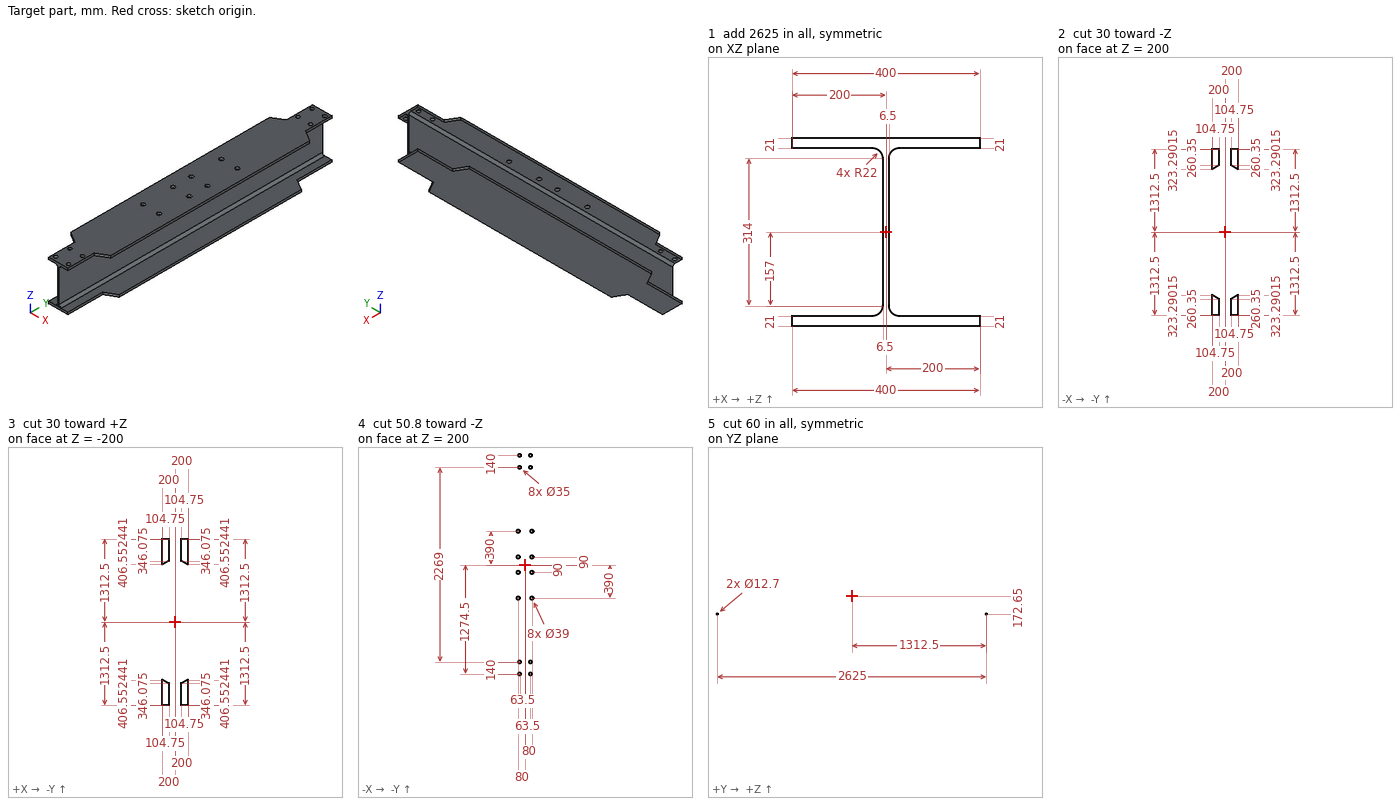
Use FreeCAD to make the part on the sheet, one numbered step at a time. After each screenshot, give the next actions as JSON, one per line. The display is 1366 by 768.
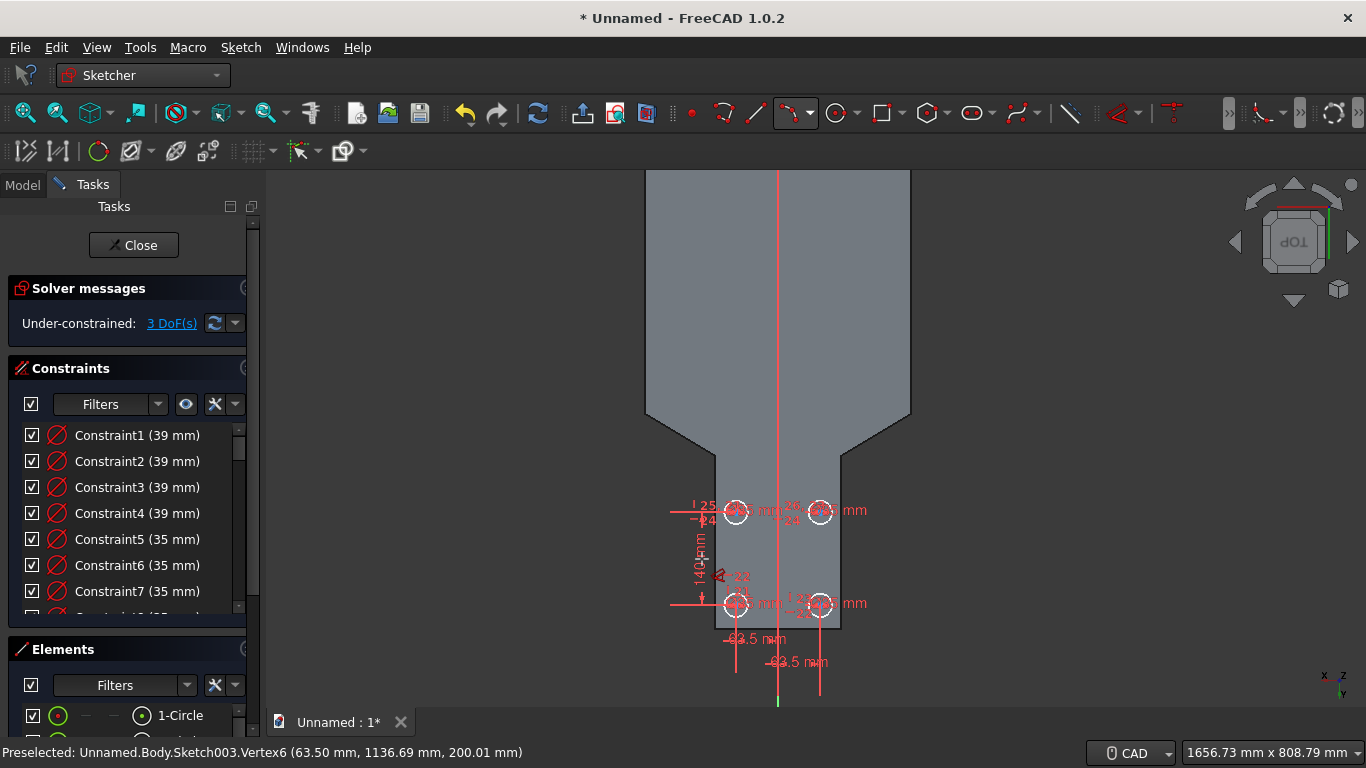
{"action": "scroll", "coordinate": [740, 611], "scroll_direction": "down", "scroll_amount": 8}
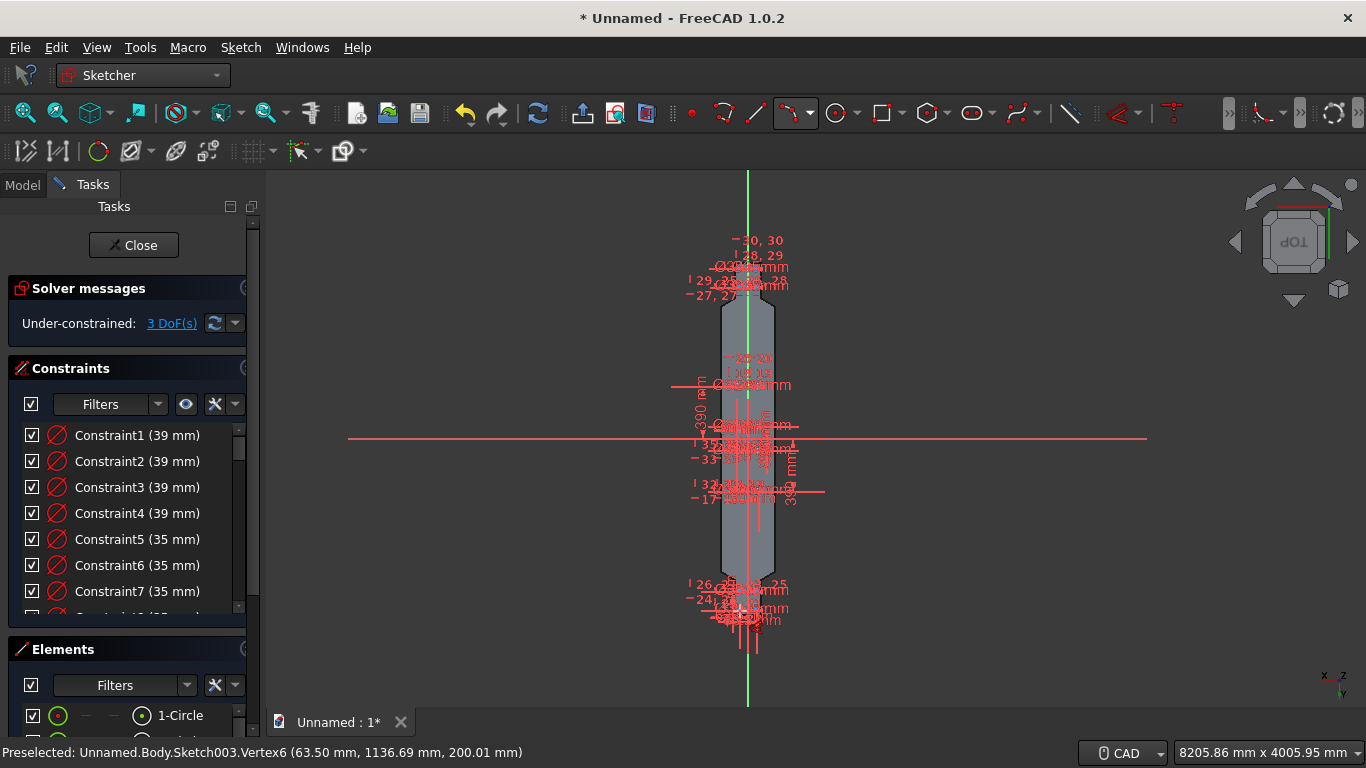
{"action": "scroll", "coordinate": [740, 288], "scroll_direction": "up", "scroll_amount": 4}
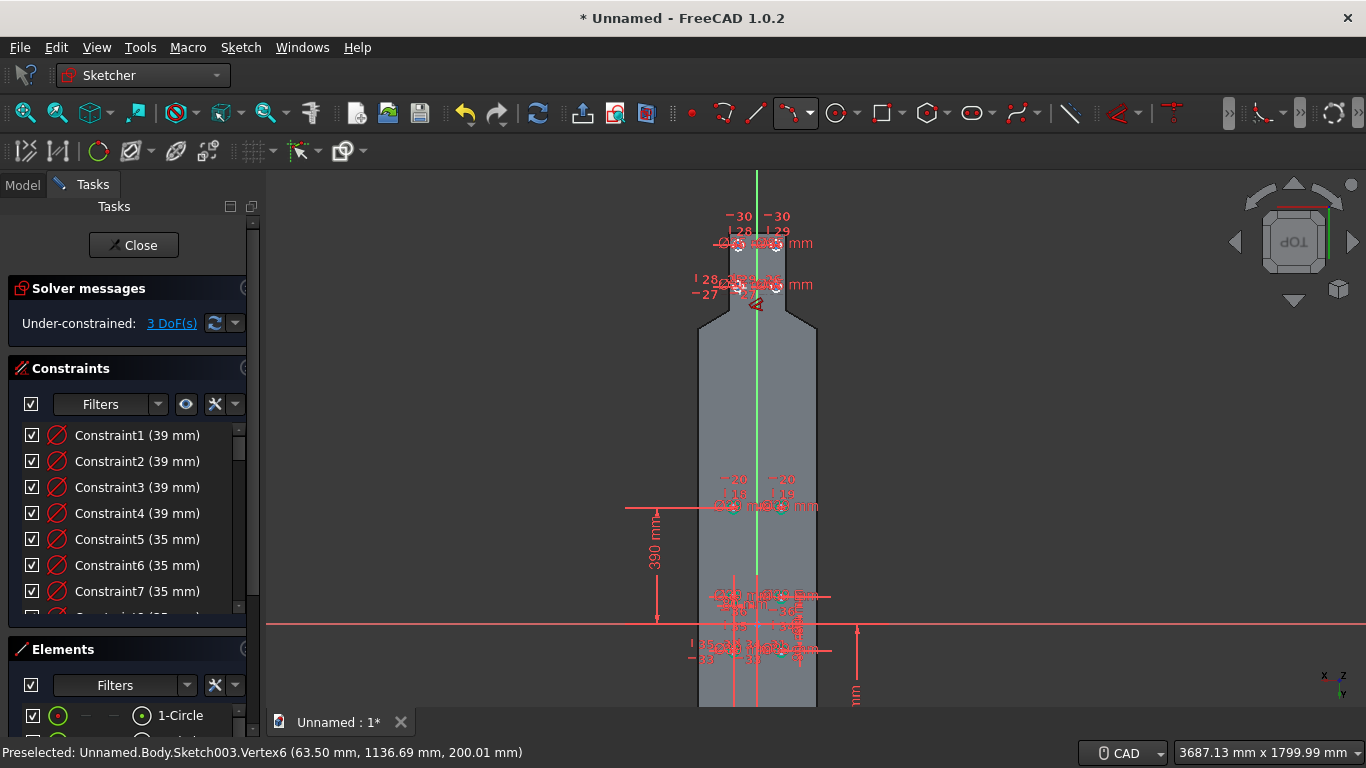
{"action": "left_click", "coordinate": [738, 287]}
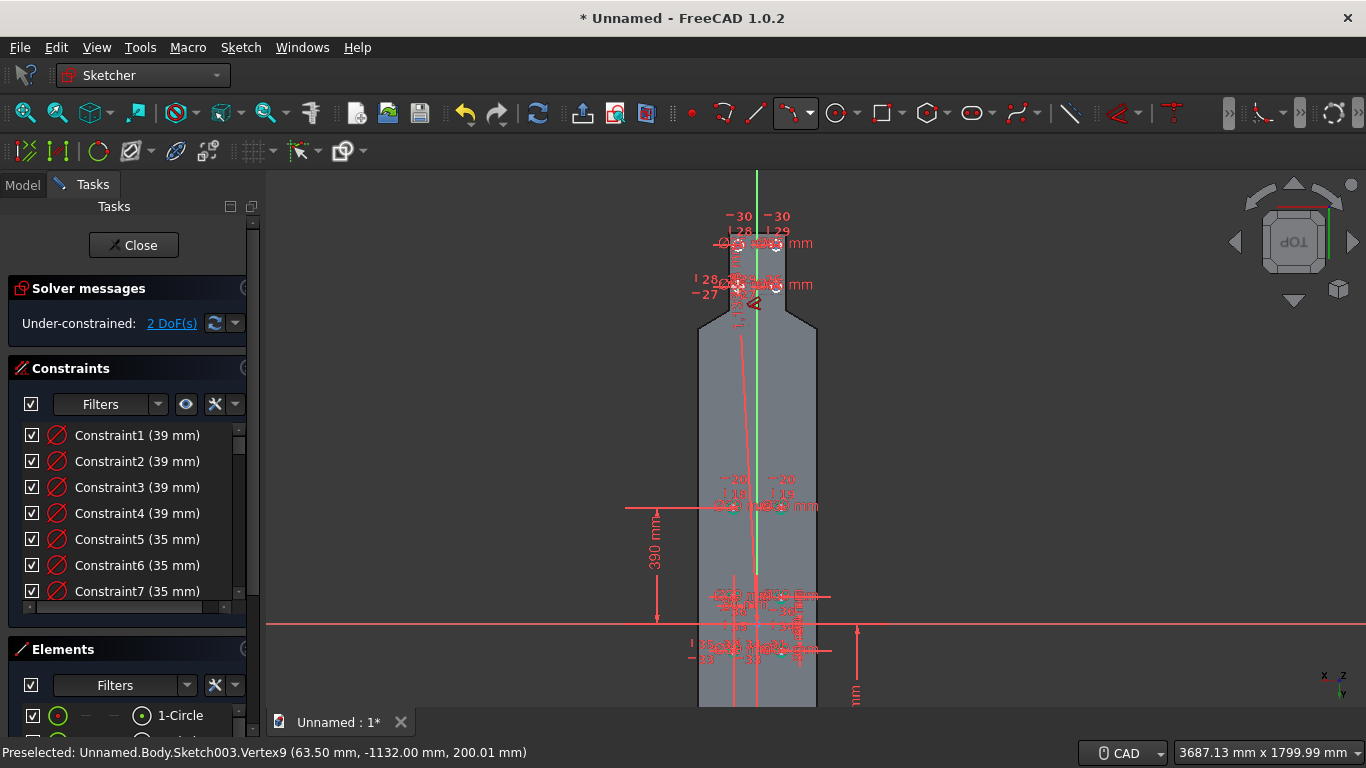
{"action": "left_click", "coordinate": [738, 245]}
{"action": "left_click", "coordinate": [704, 266]}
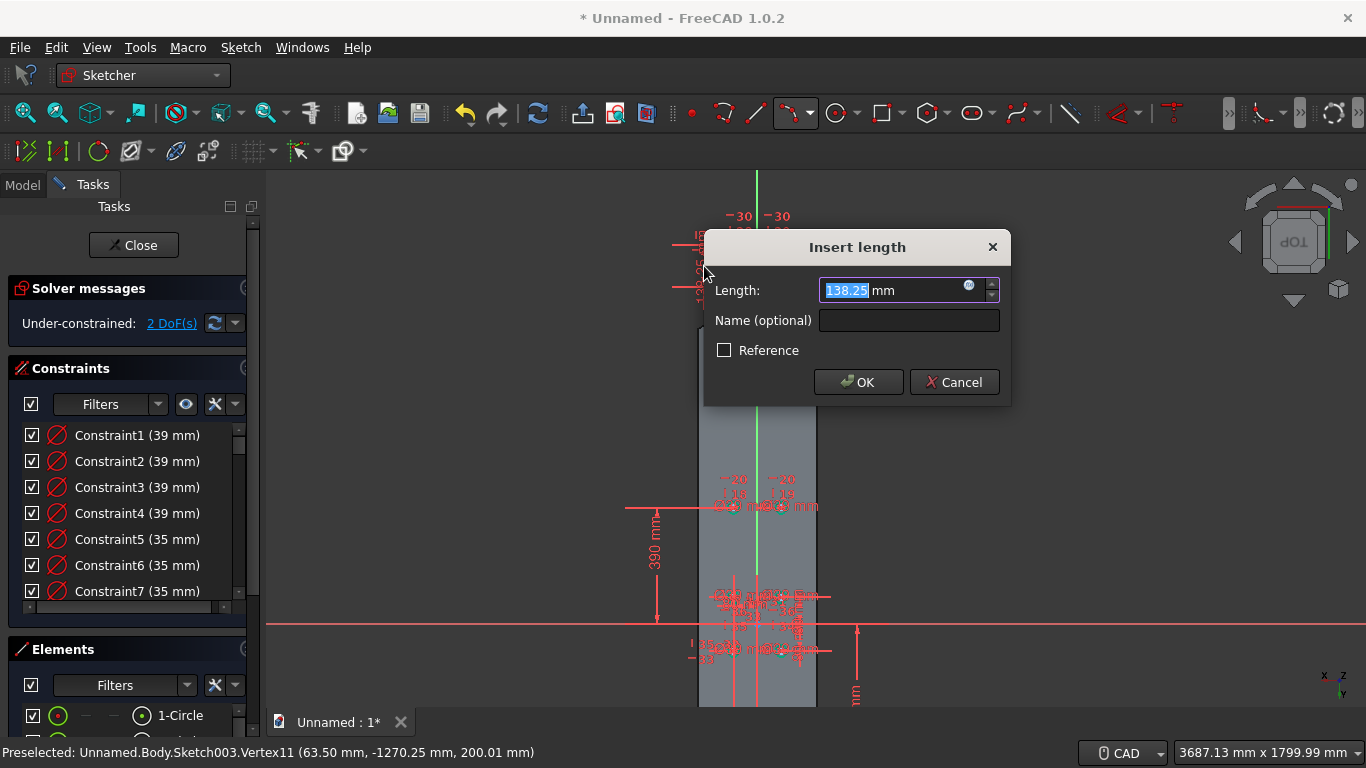
{"action": "type", "text": "140"}
{"action": "key", "text": "Return"}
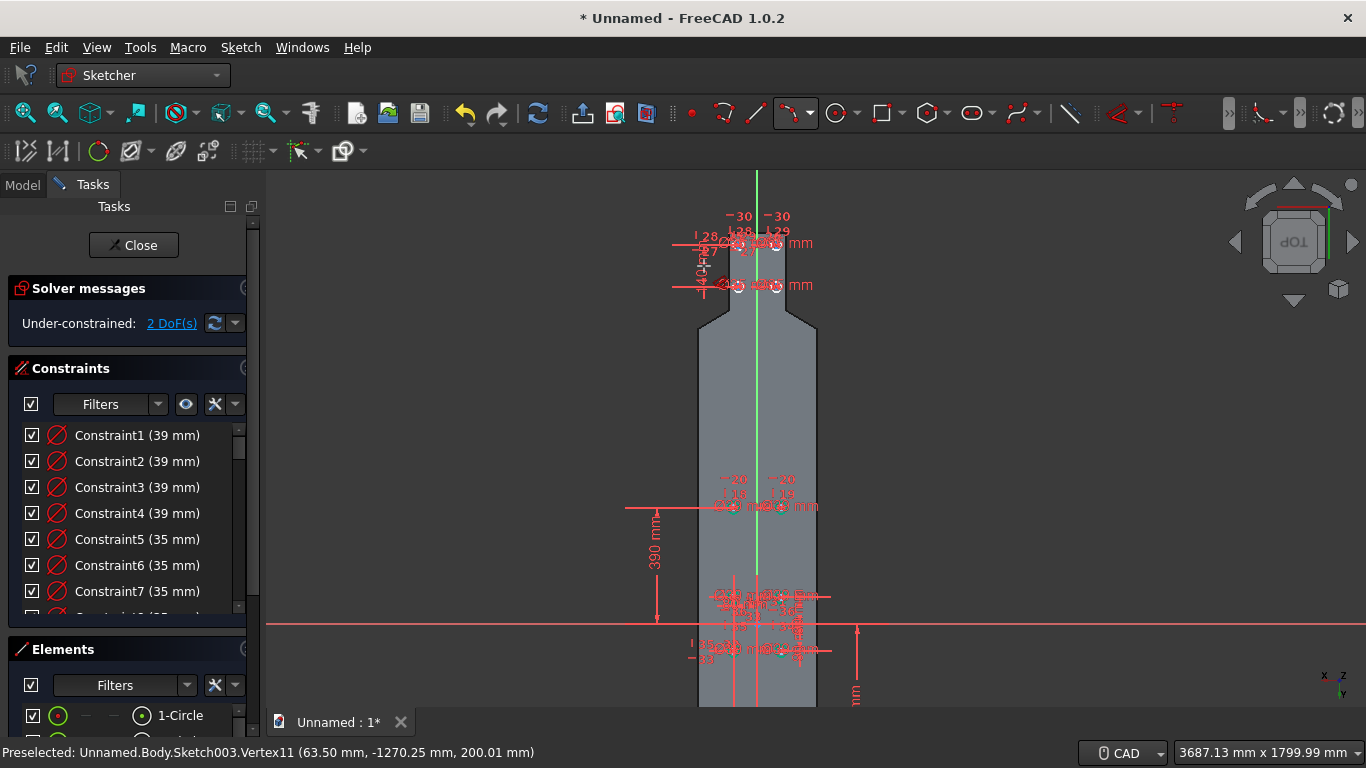
{"action": "scroll", "coordinate": [739, 287], "scroll_direction": "down", "scroll_amount": 4}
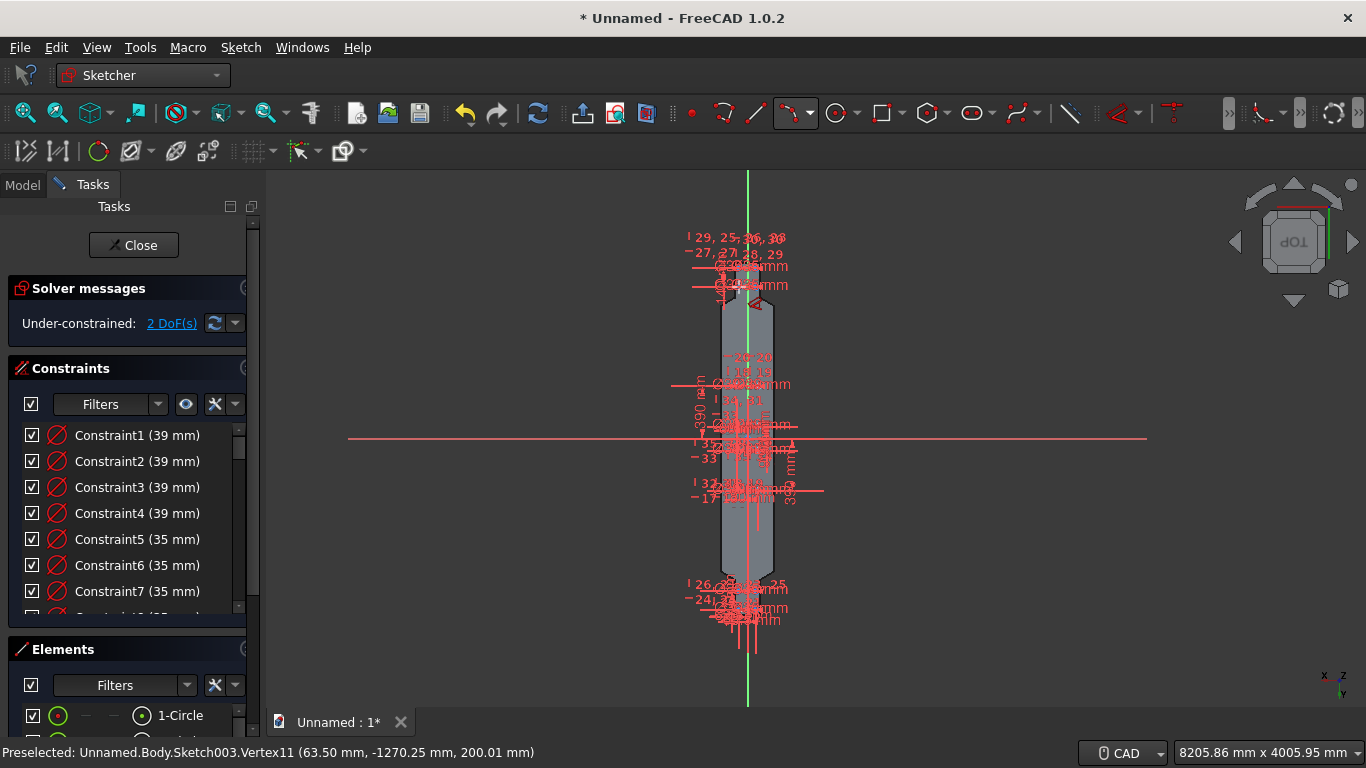
{"action": "left_click", "coordinate": [739, 591]}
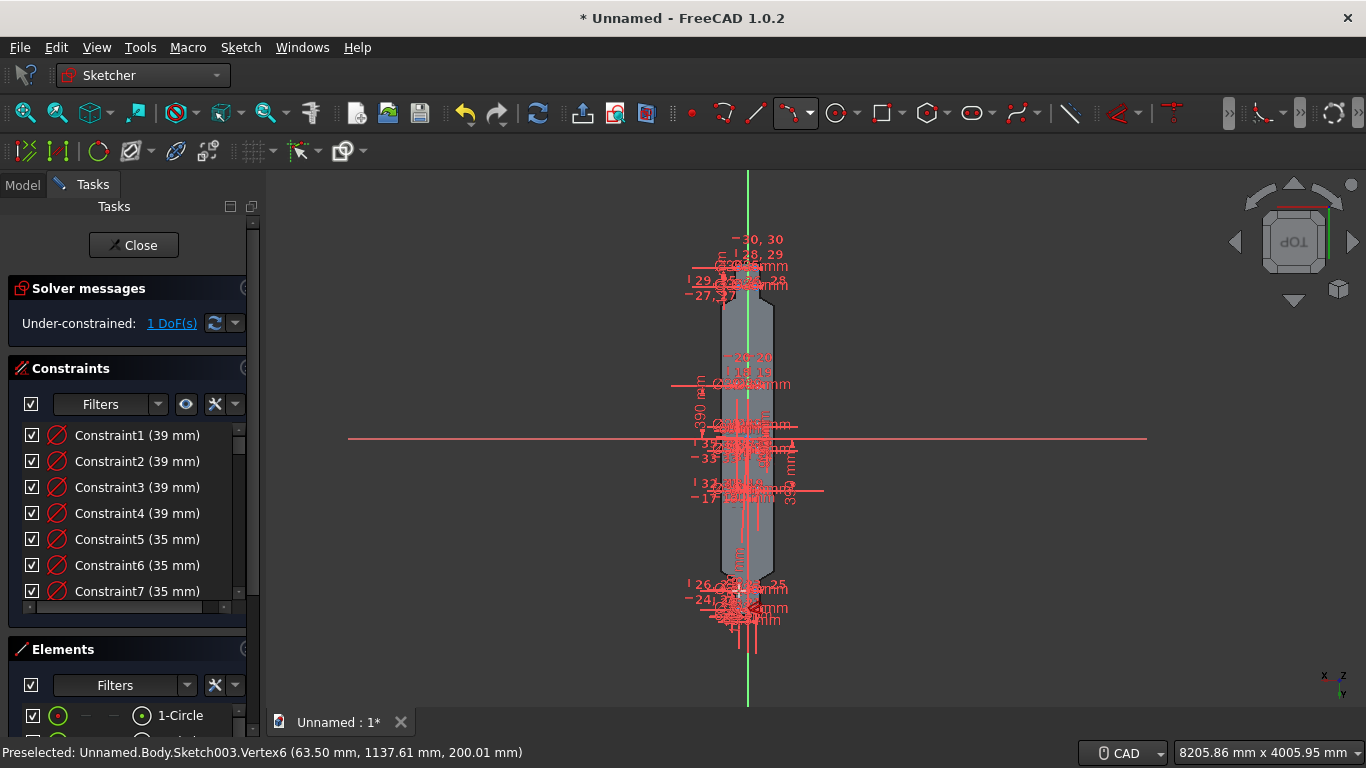
{"action": "left_click", "coordinate": [739, 287]}
{"action": "left_click", "coordinate": [705, 369]}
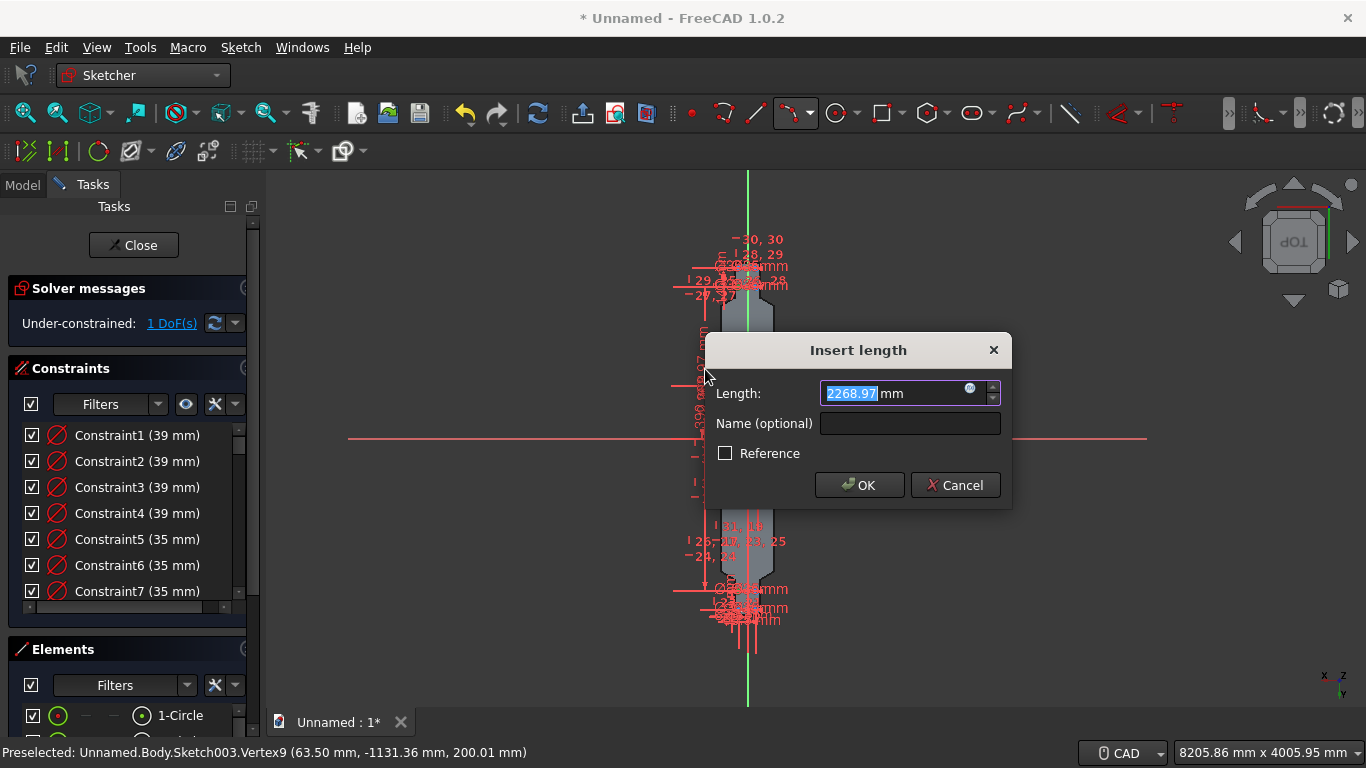
{"action": "type", "text": "2269"}
{"action": "key", "text": "Return"}